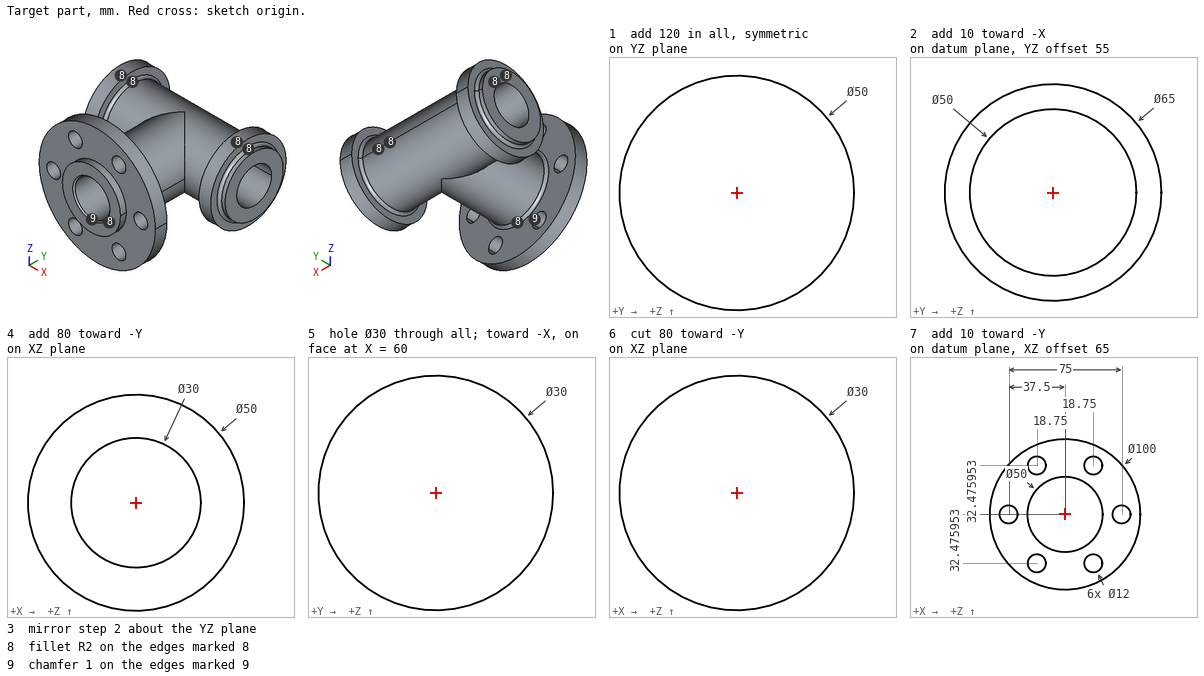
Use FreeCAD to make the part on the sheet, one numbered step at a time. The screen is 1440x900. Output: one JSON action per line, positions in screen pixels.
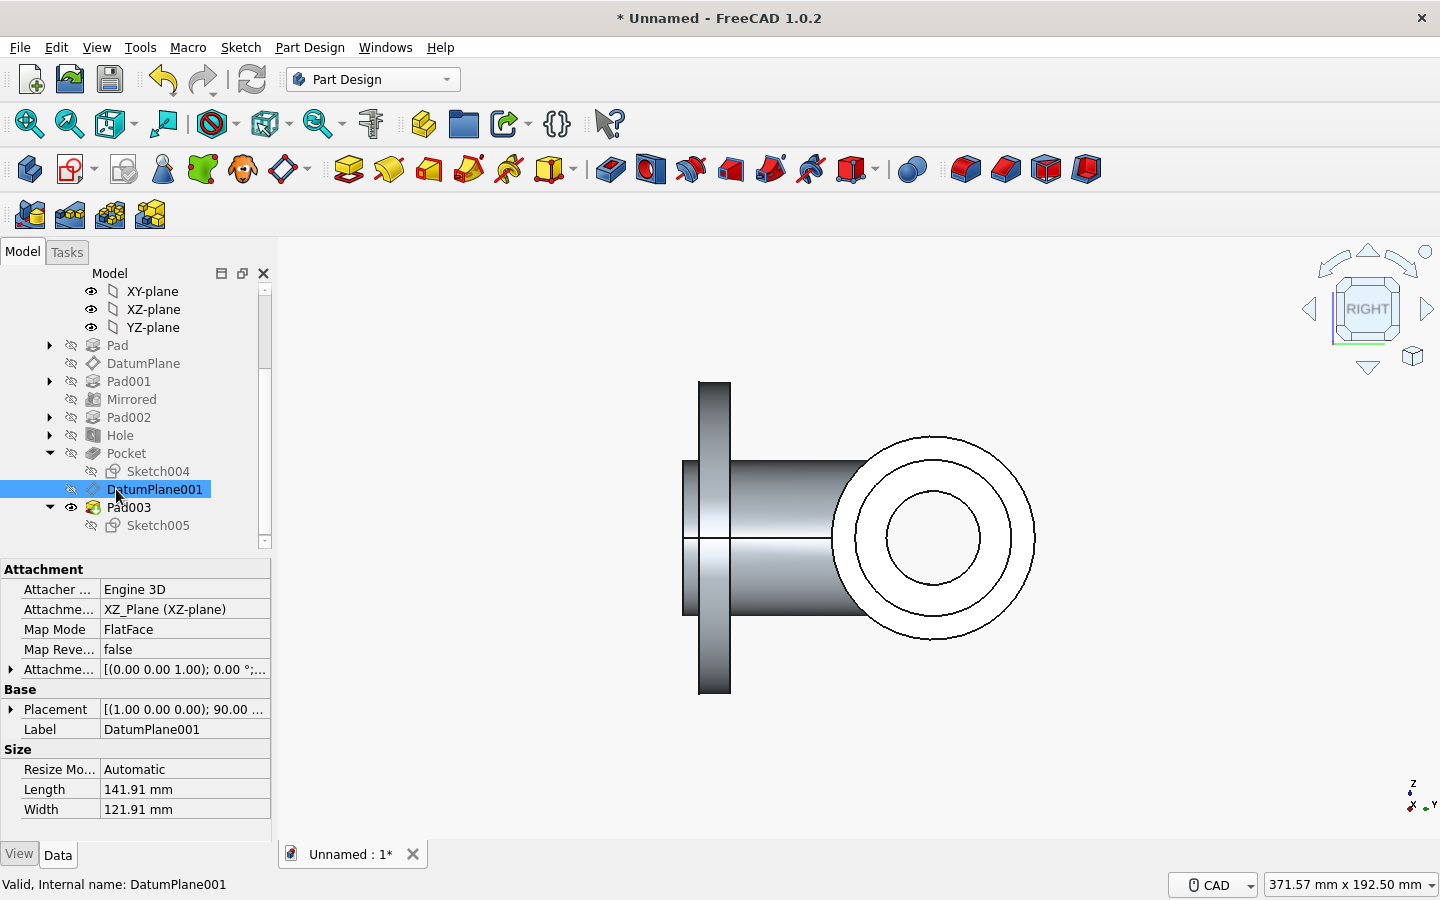
{"action": "key", "text": "5"}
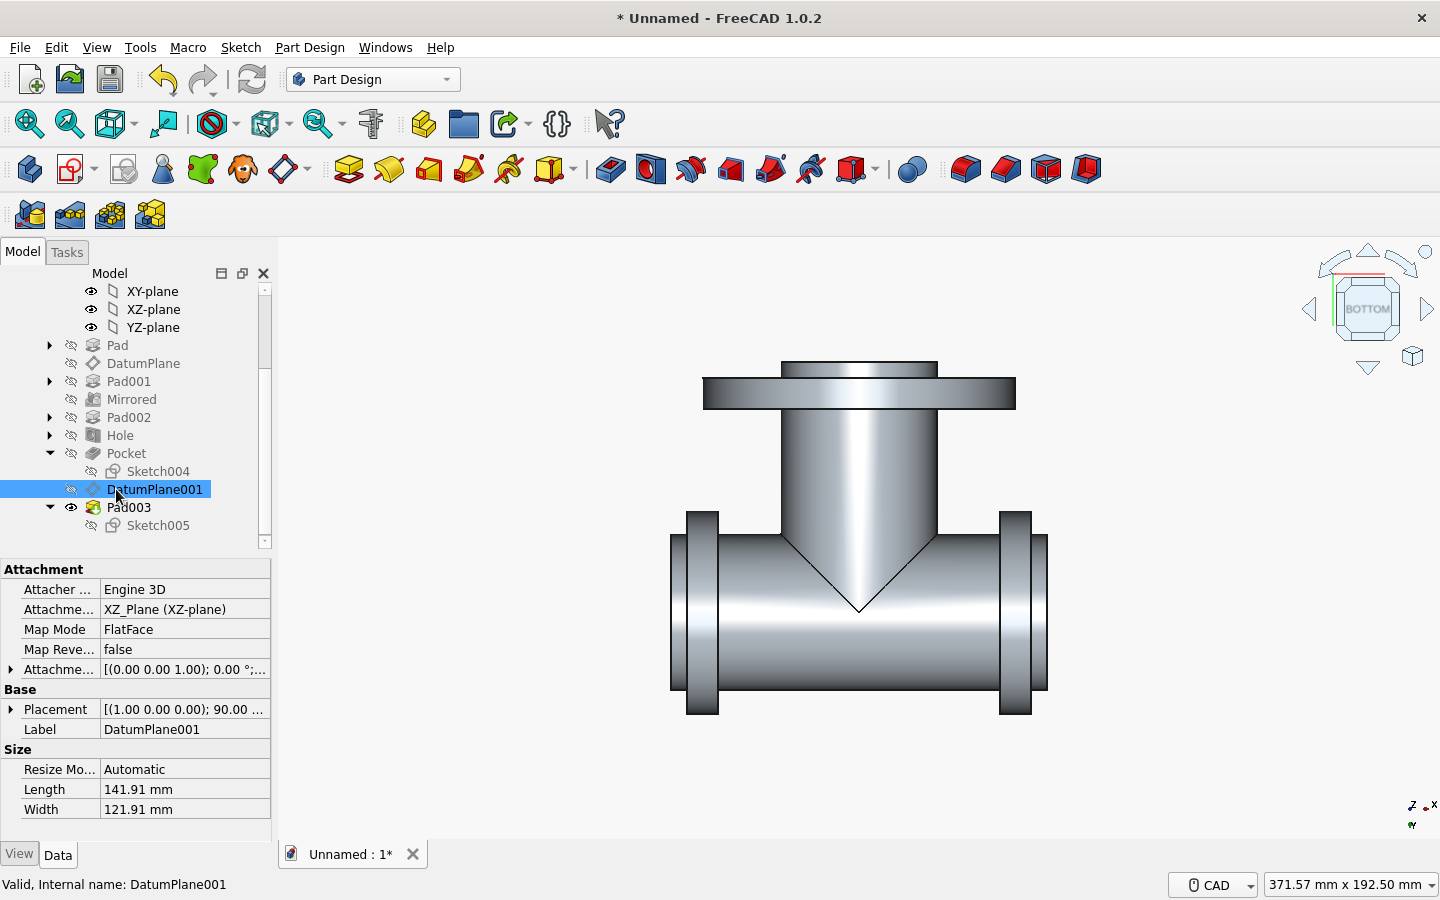
{"action": "key", "text": "4"}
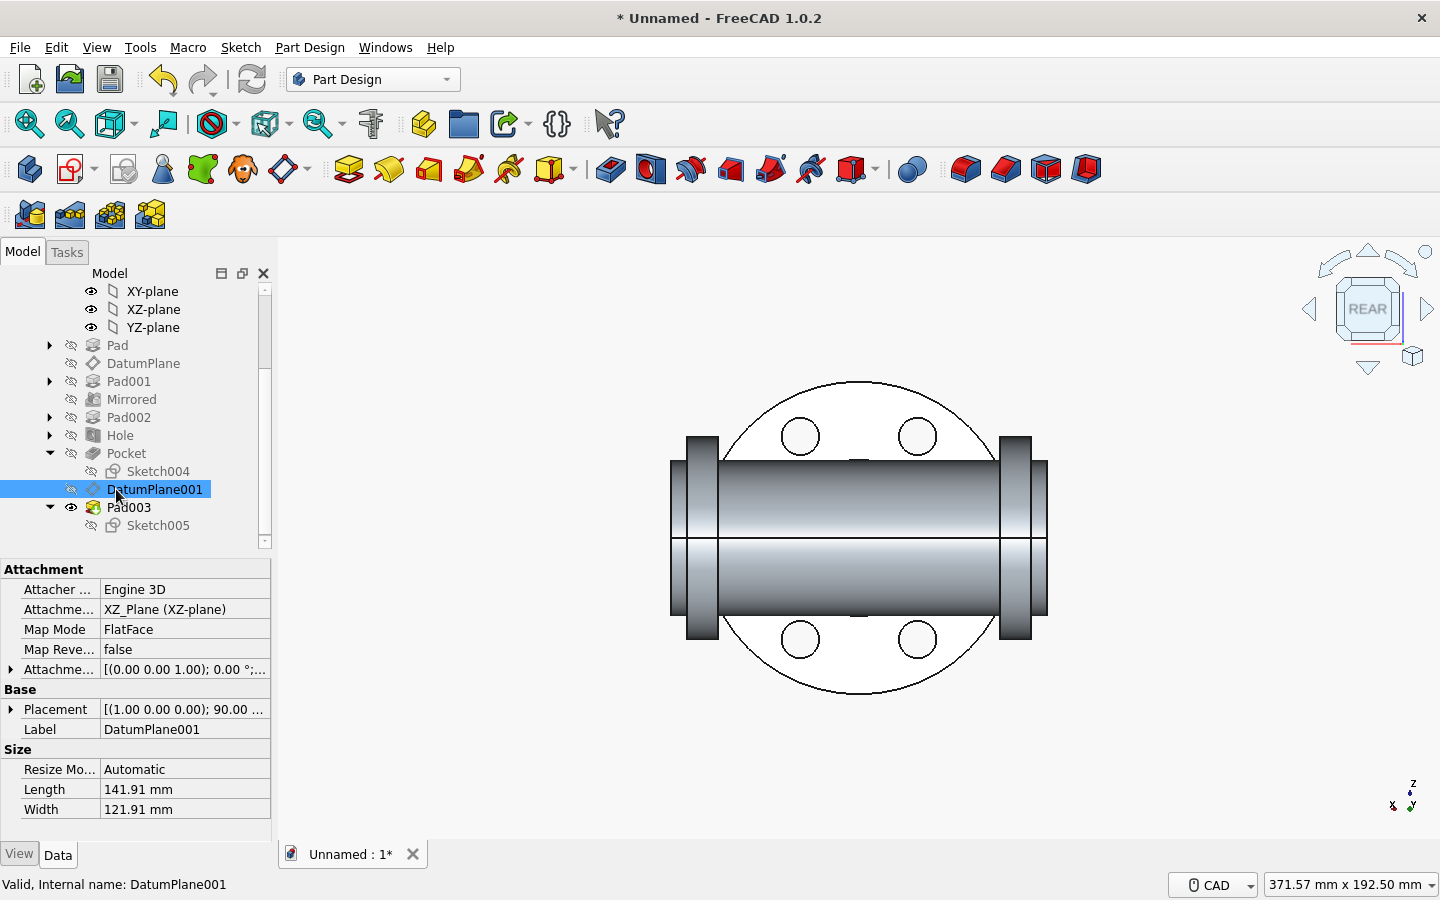
{"action": "key", "text": "6"}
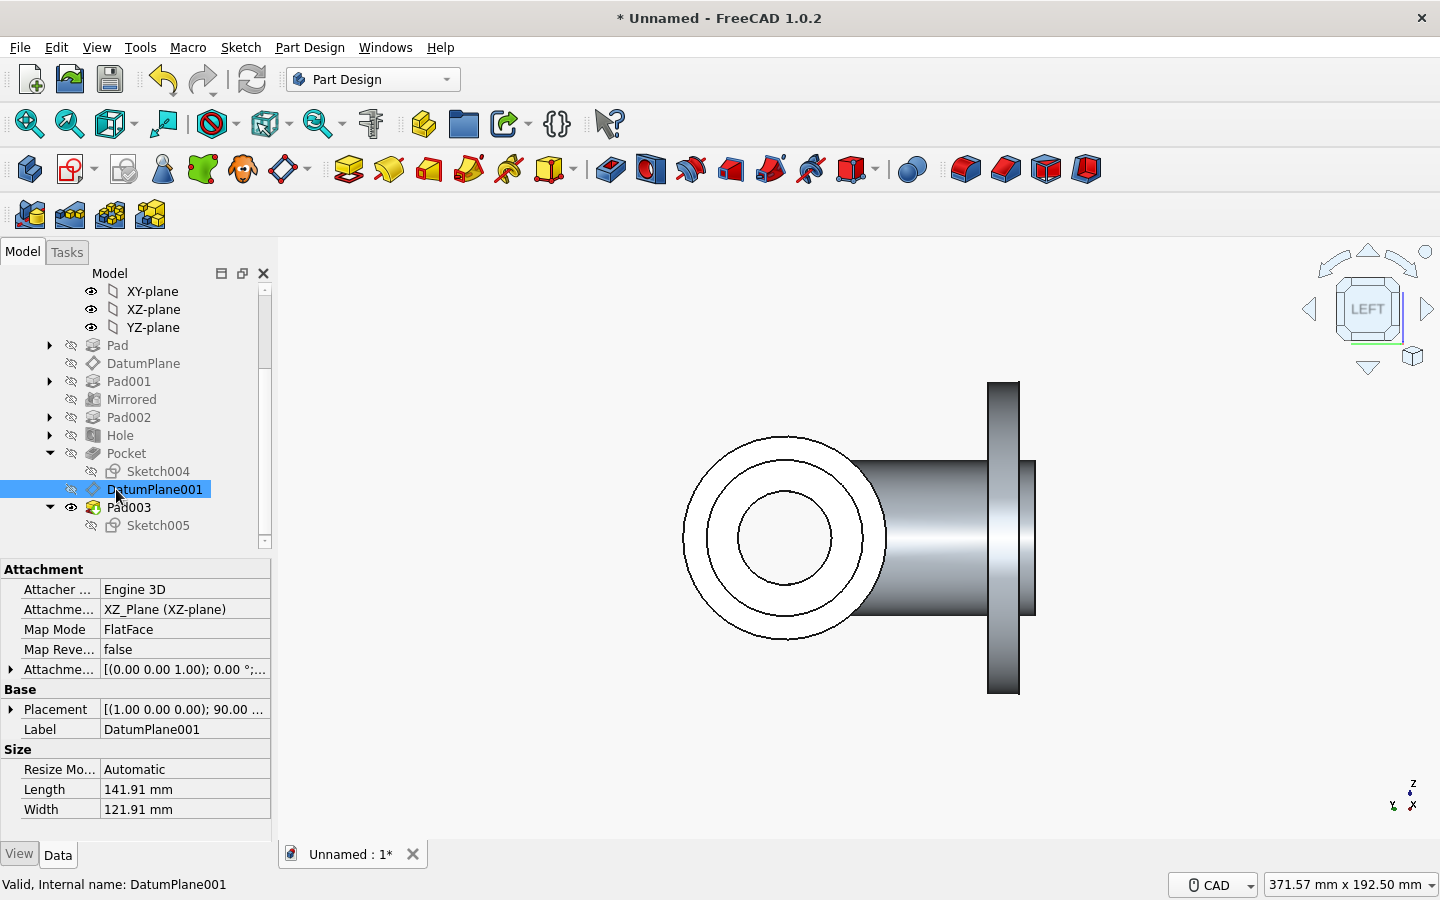
{"action": "key", "text": "v 3"}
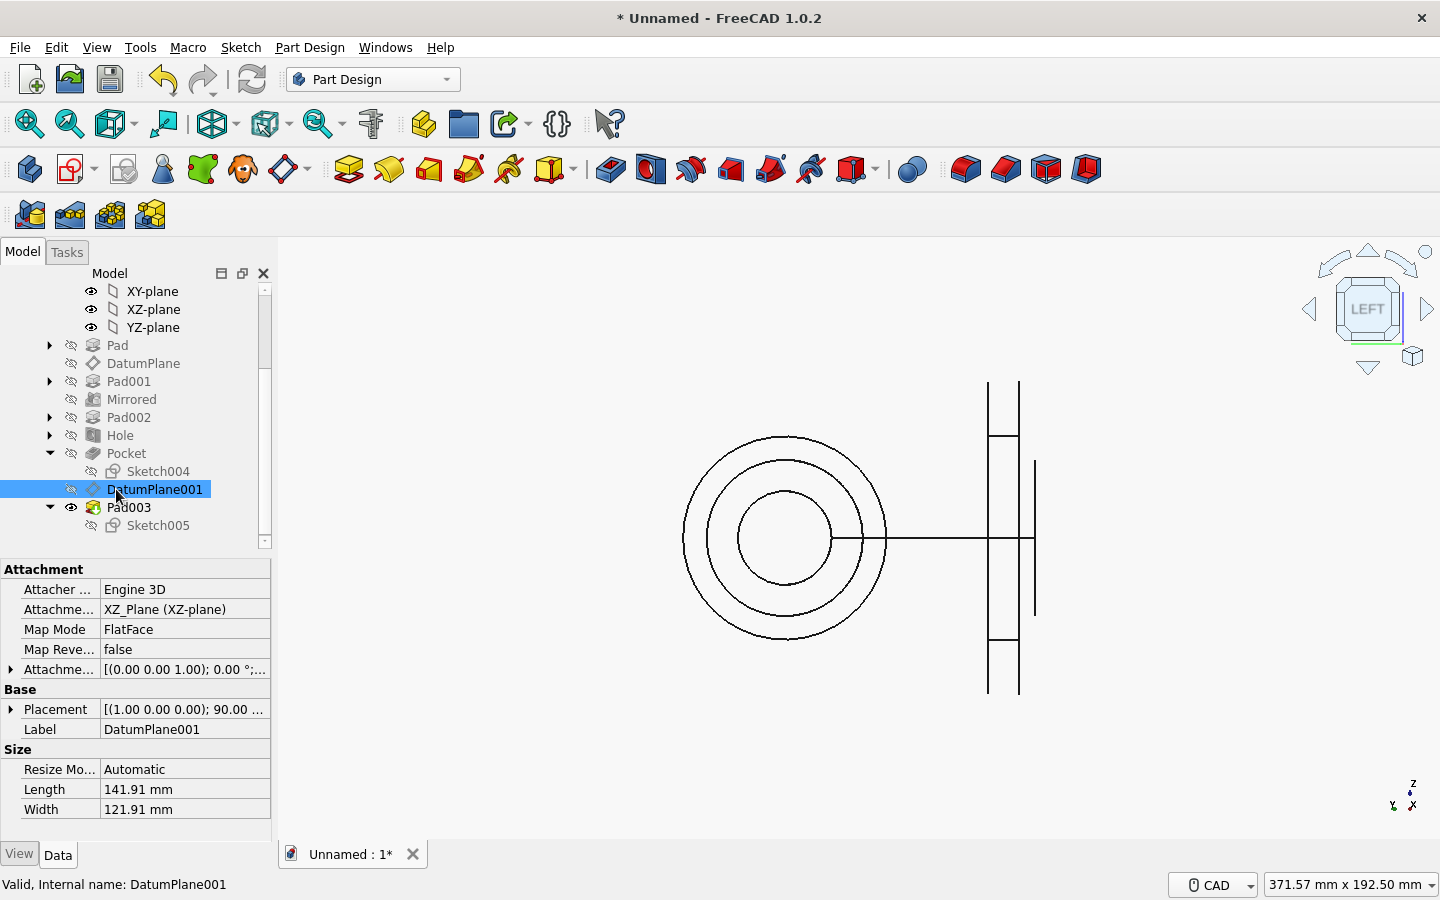
{"action": "key", "text": "0"}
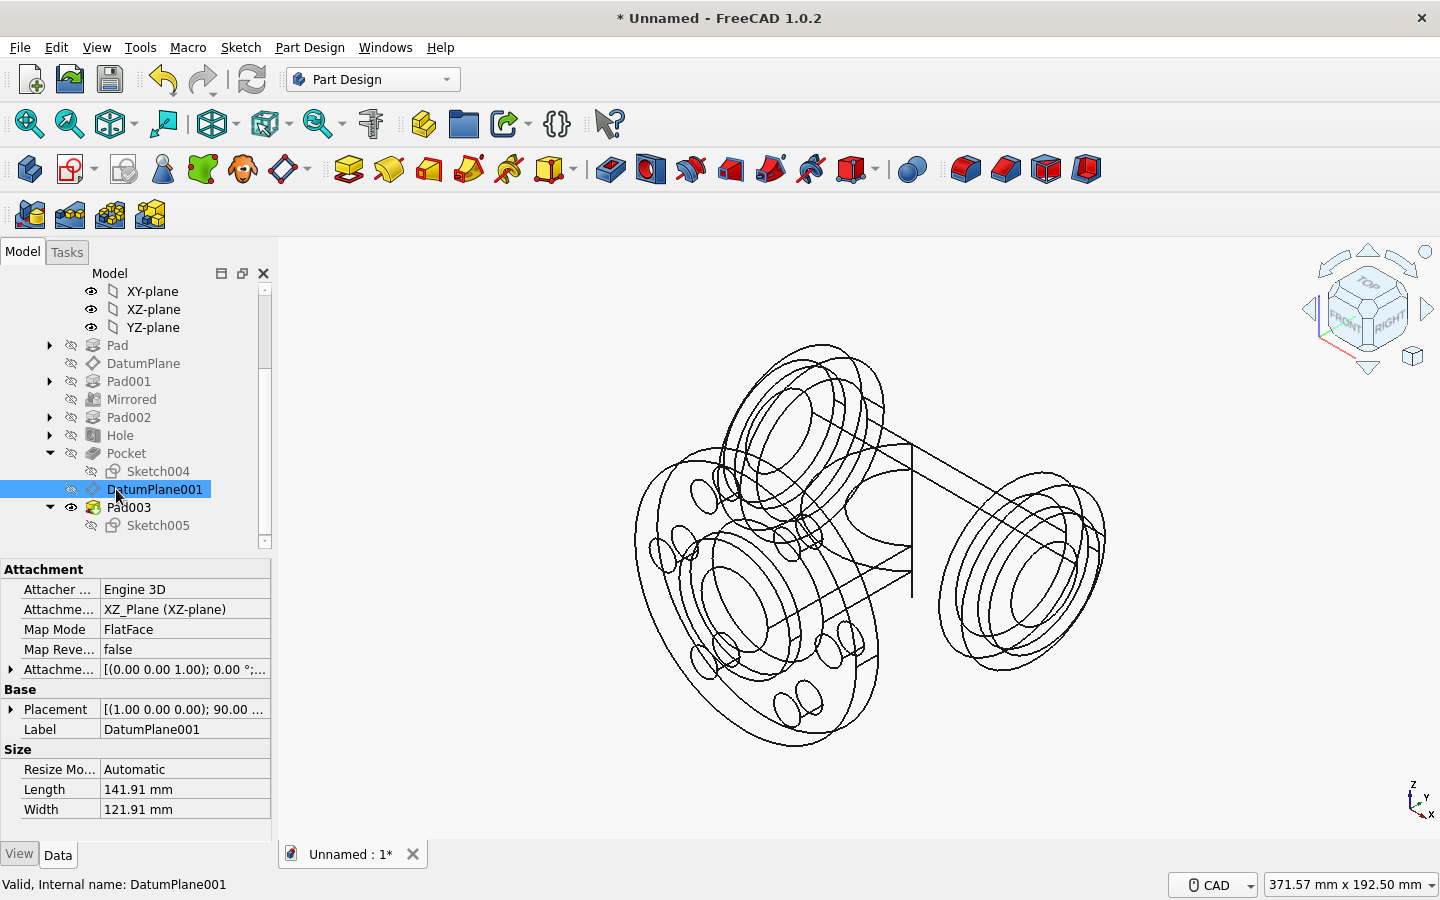
{"action": "left_click", "coordinate": [767, 438]}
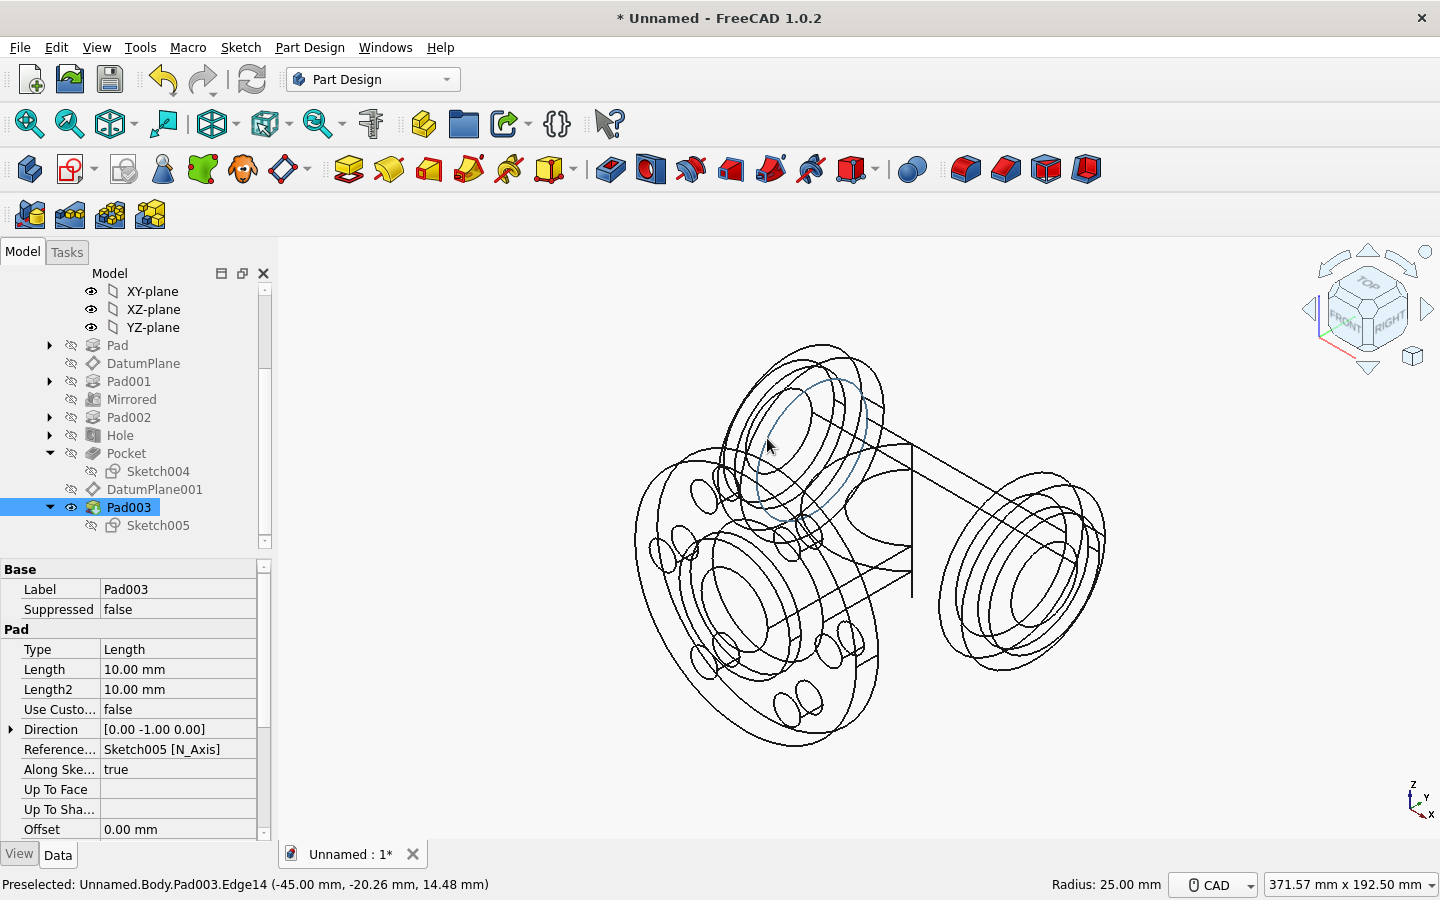
{"action": "left_click", "coordinate": [745, 425], "text": "ctrl"}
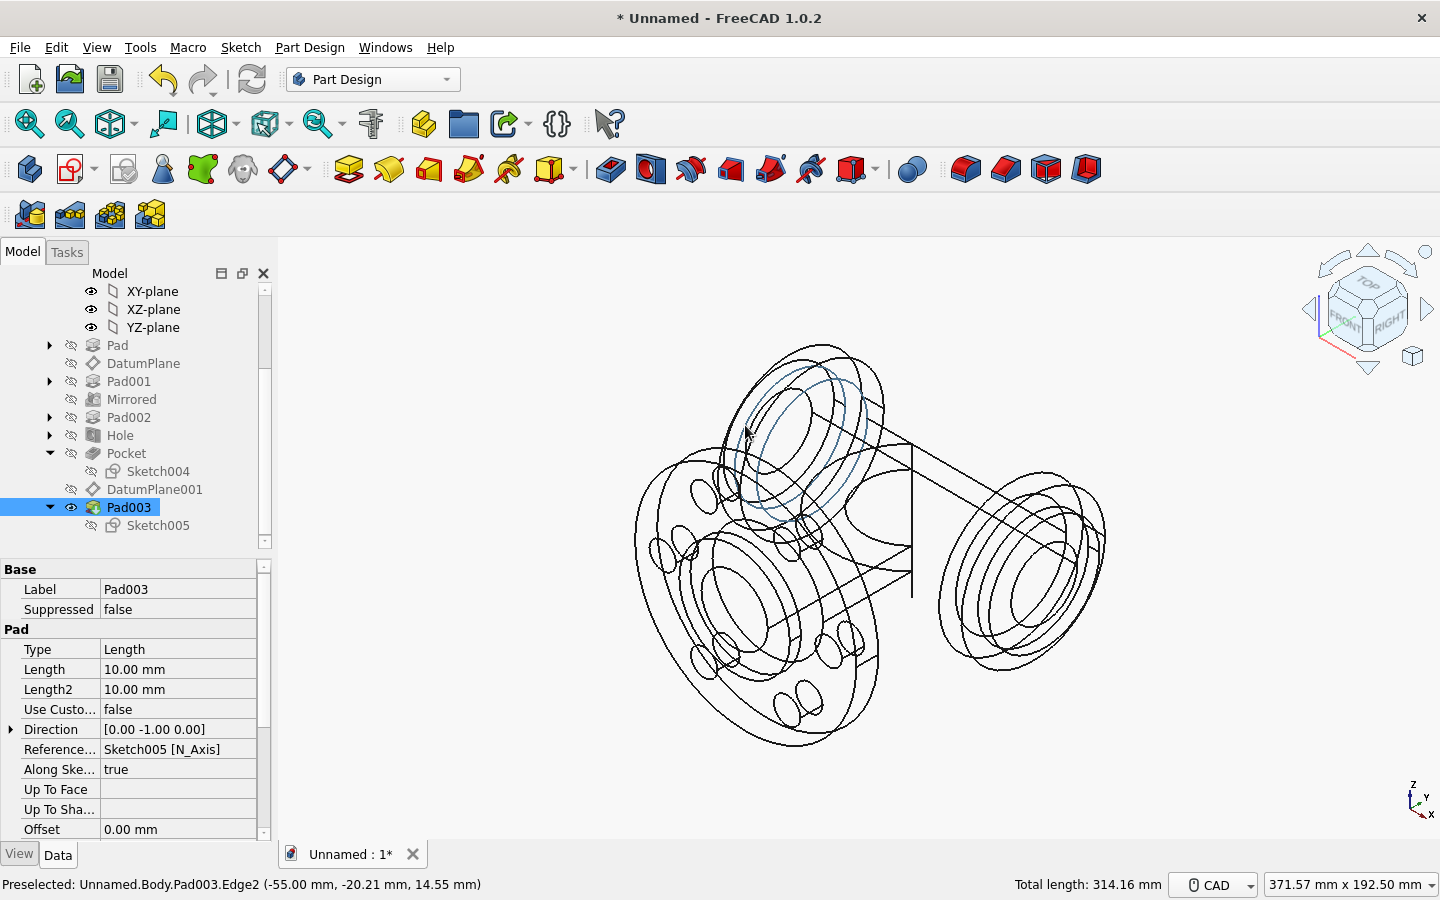
{"action": "left_click", "coordinate": [713, 558], "text": "ctrl"}